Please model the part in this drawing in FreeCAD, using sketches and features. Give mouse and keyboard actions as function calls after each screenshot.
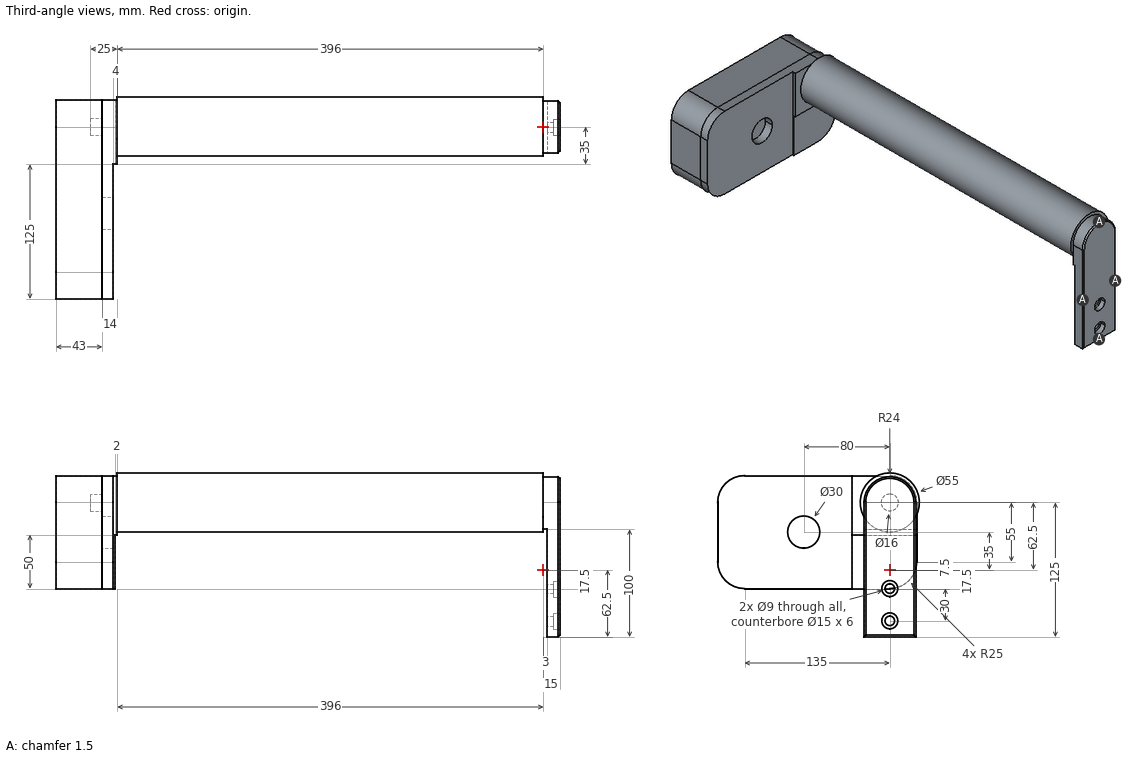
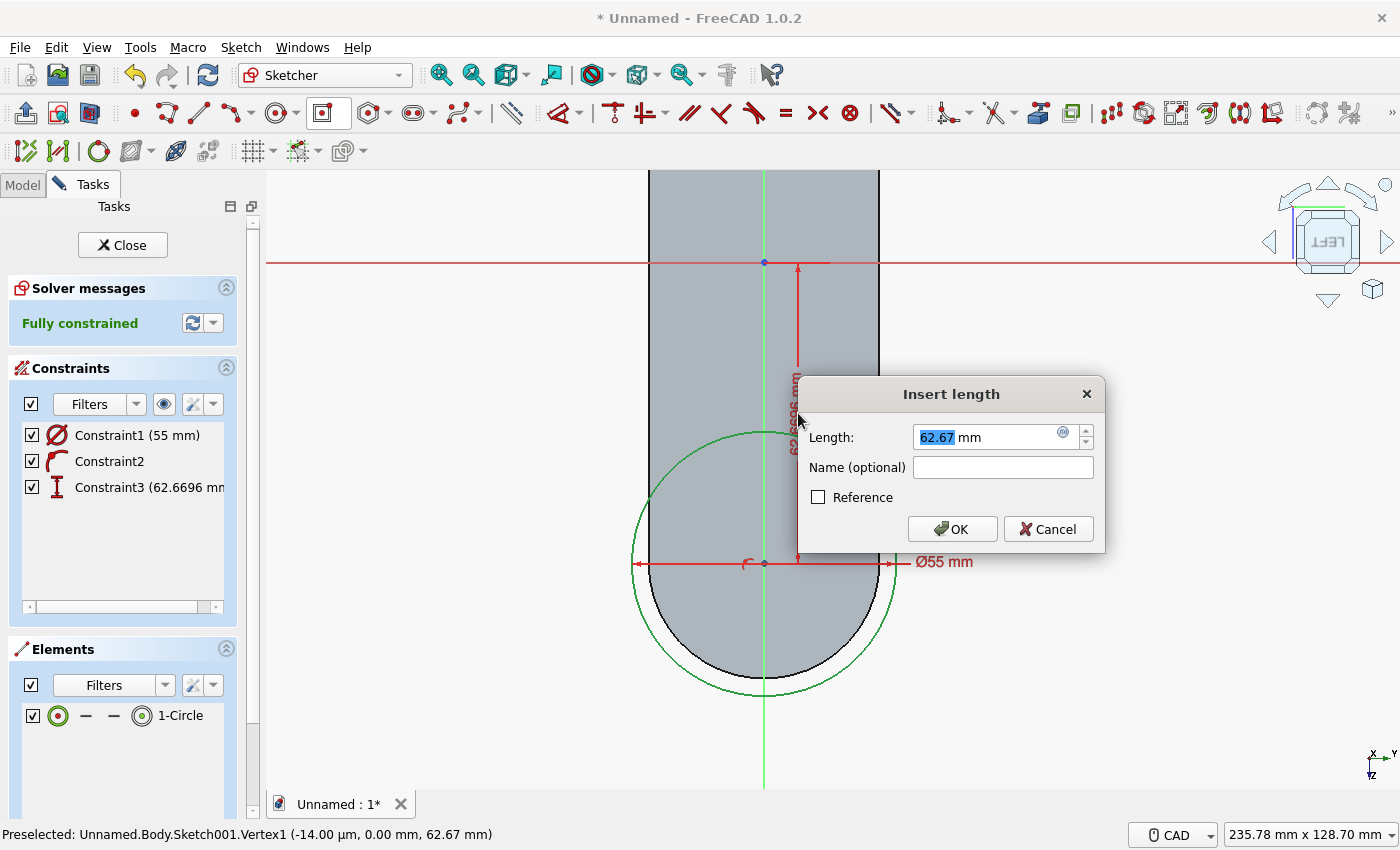
text(62.5)
key(Return)
key(Escape)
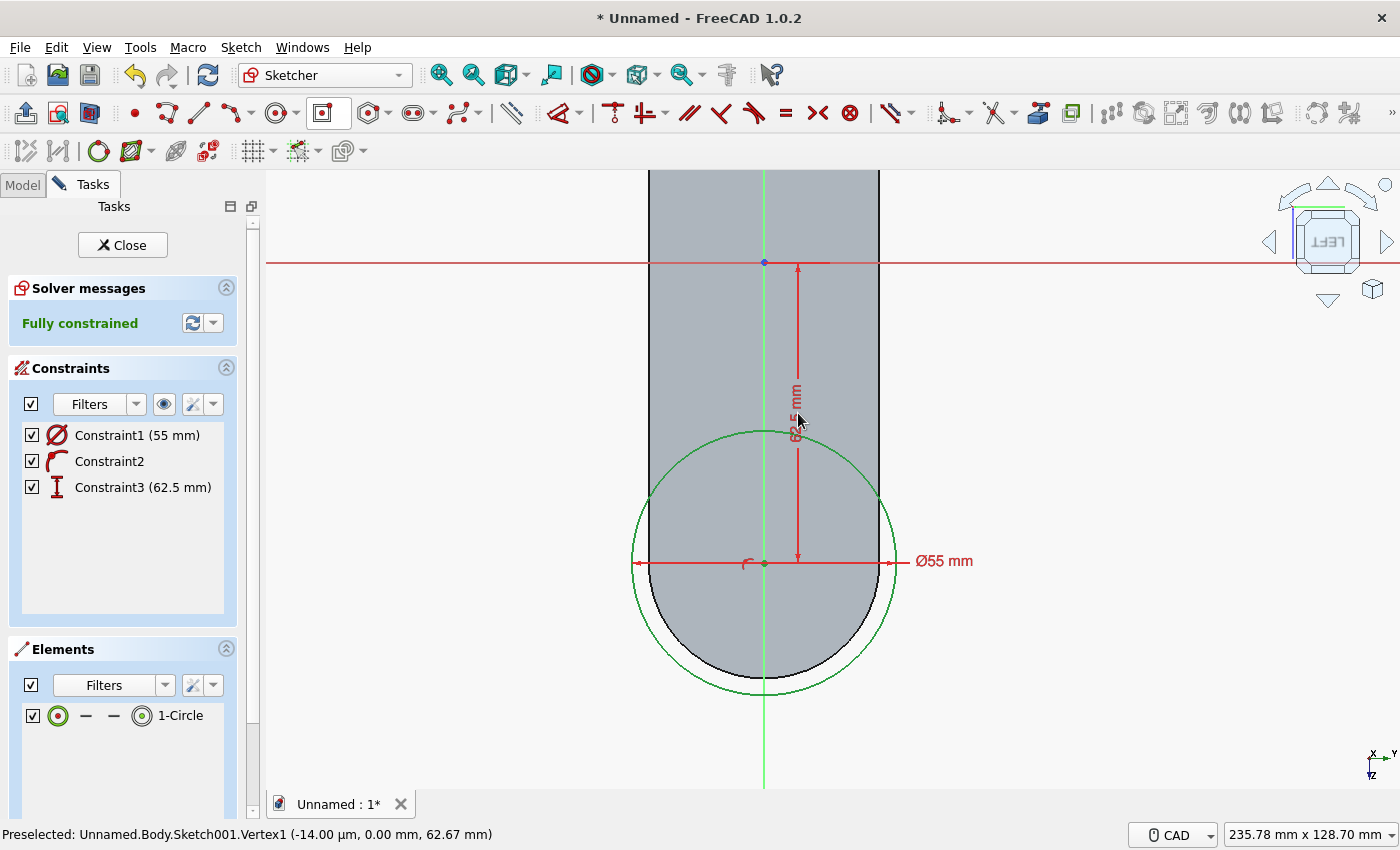
click(123, 245)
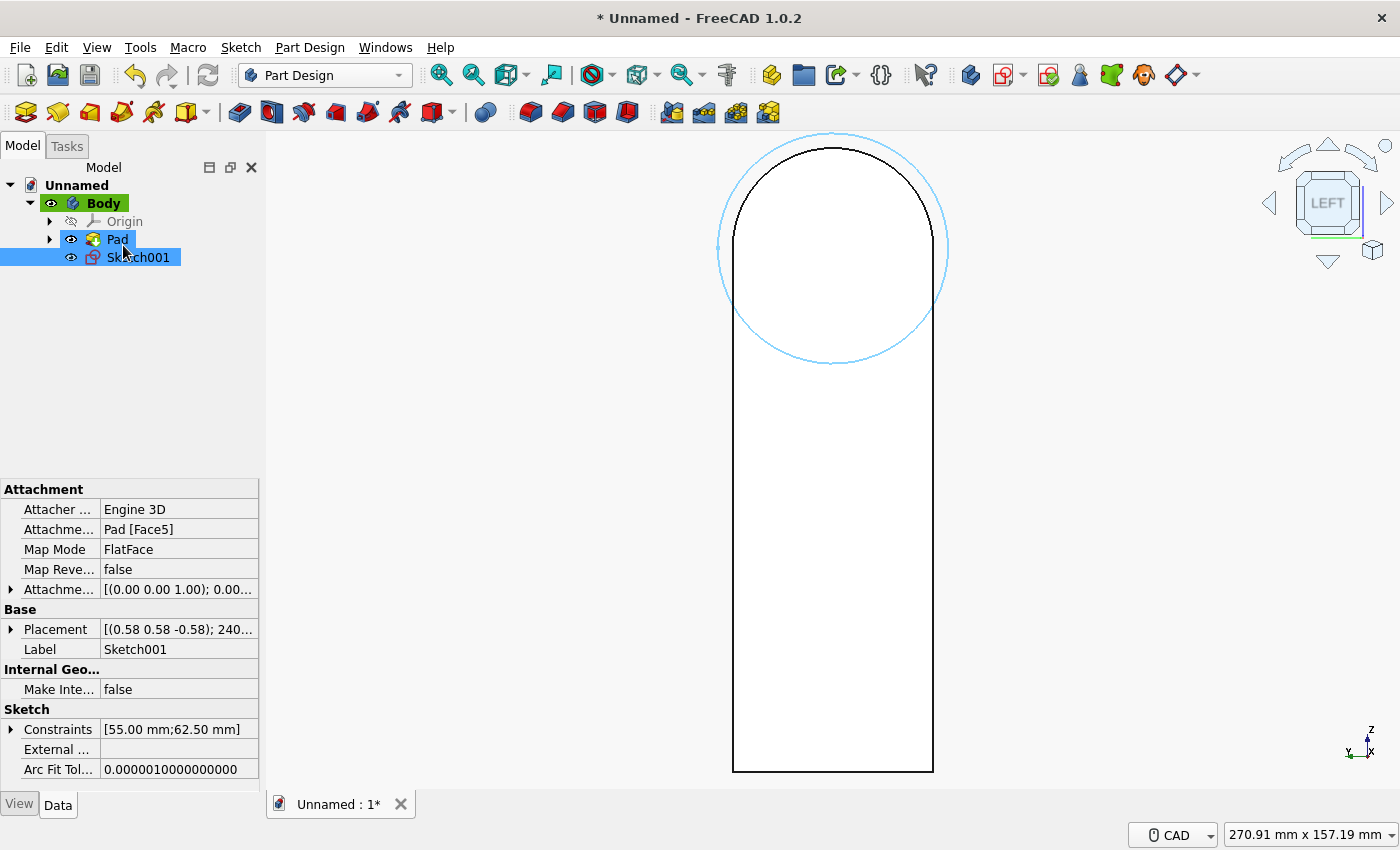
click(26, 112)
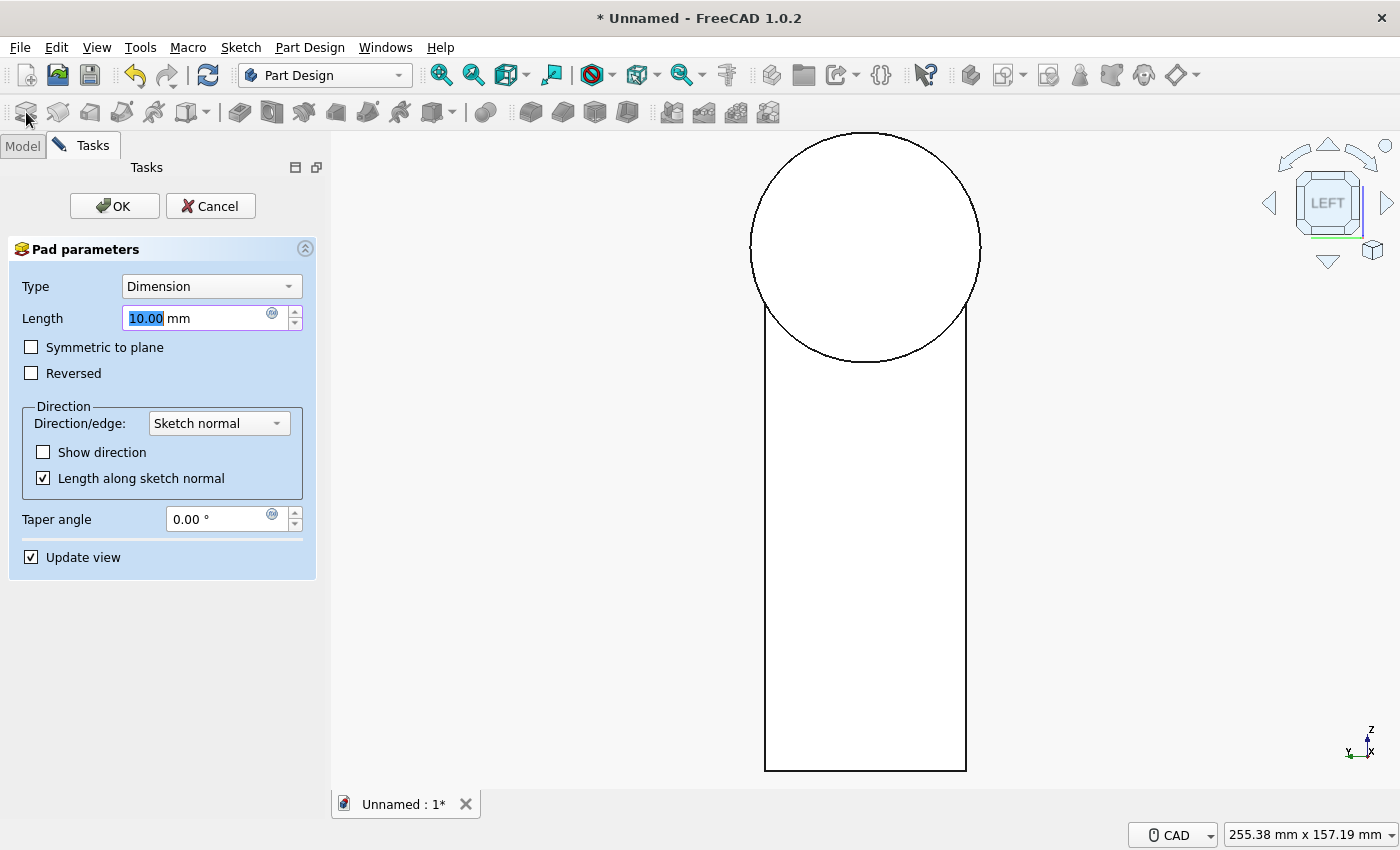
text(396)
key(Tab)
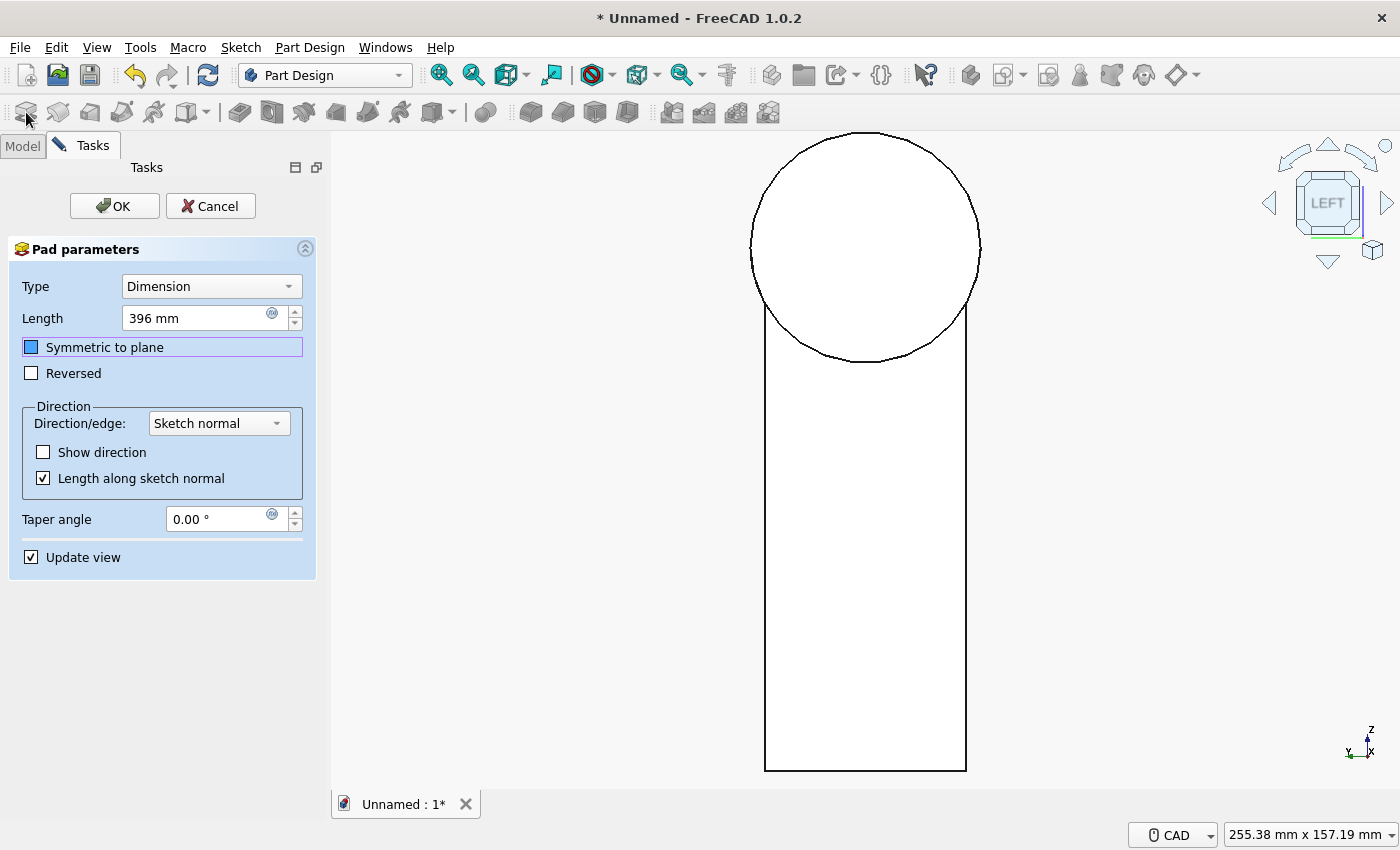
click(115, 206)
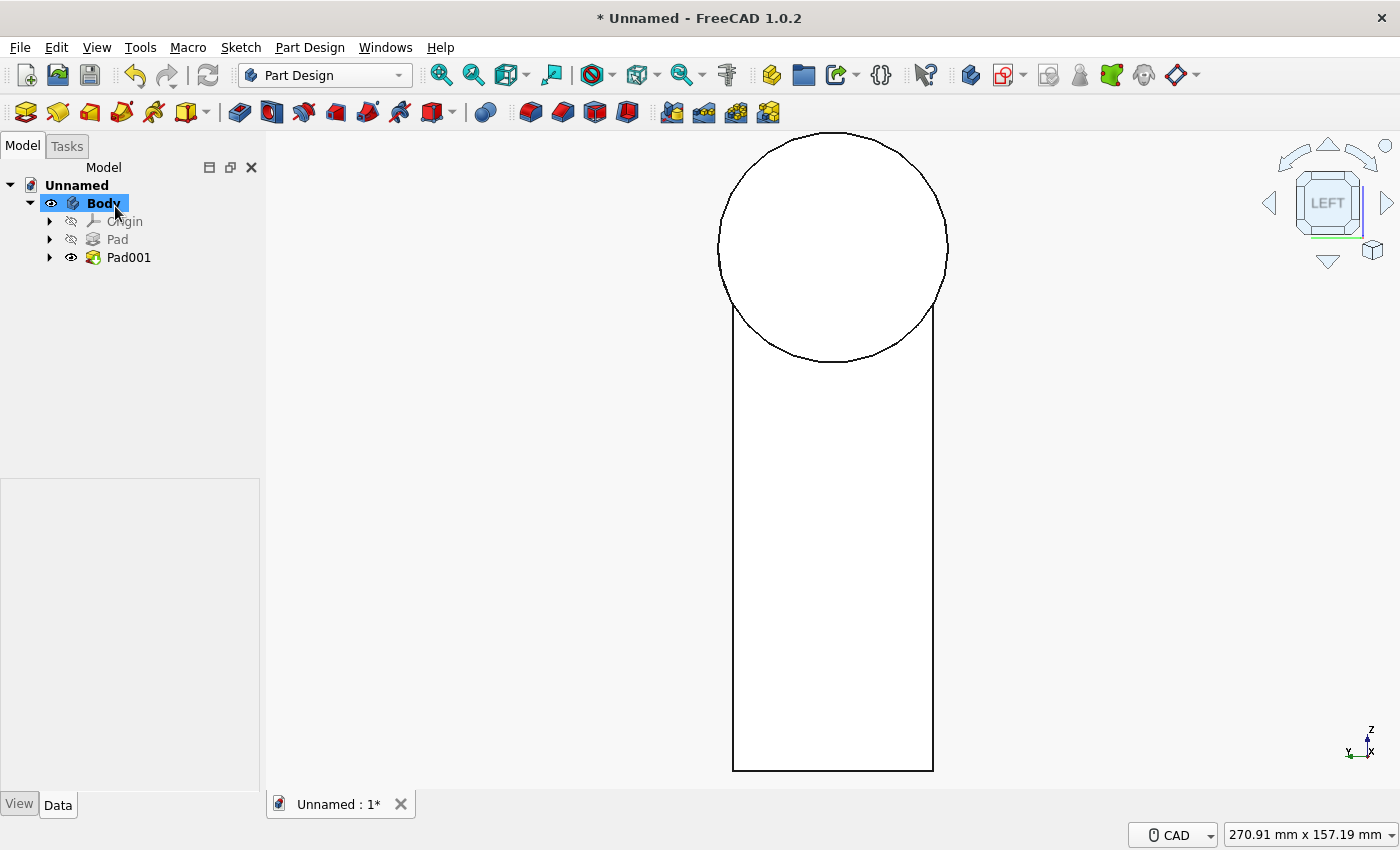
key(0)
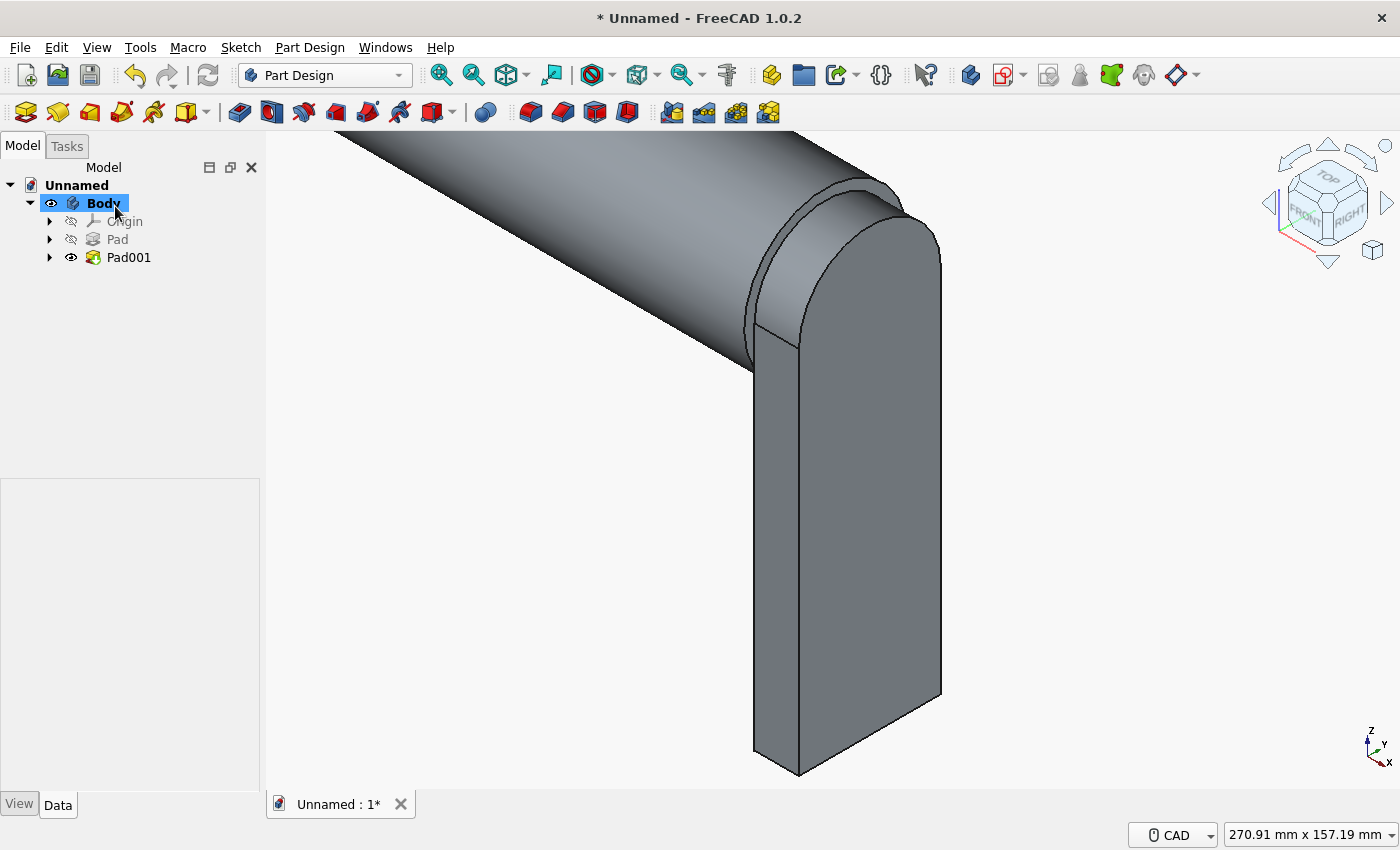
click(442, 76)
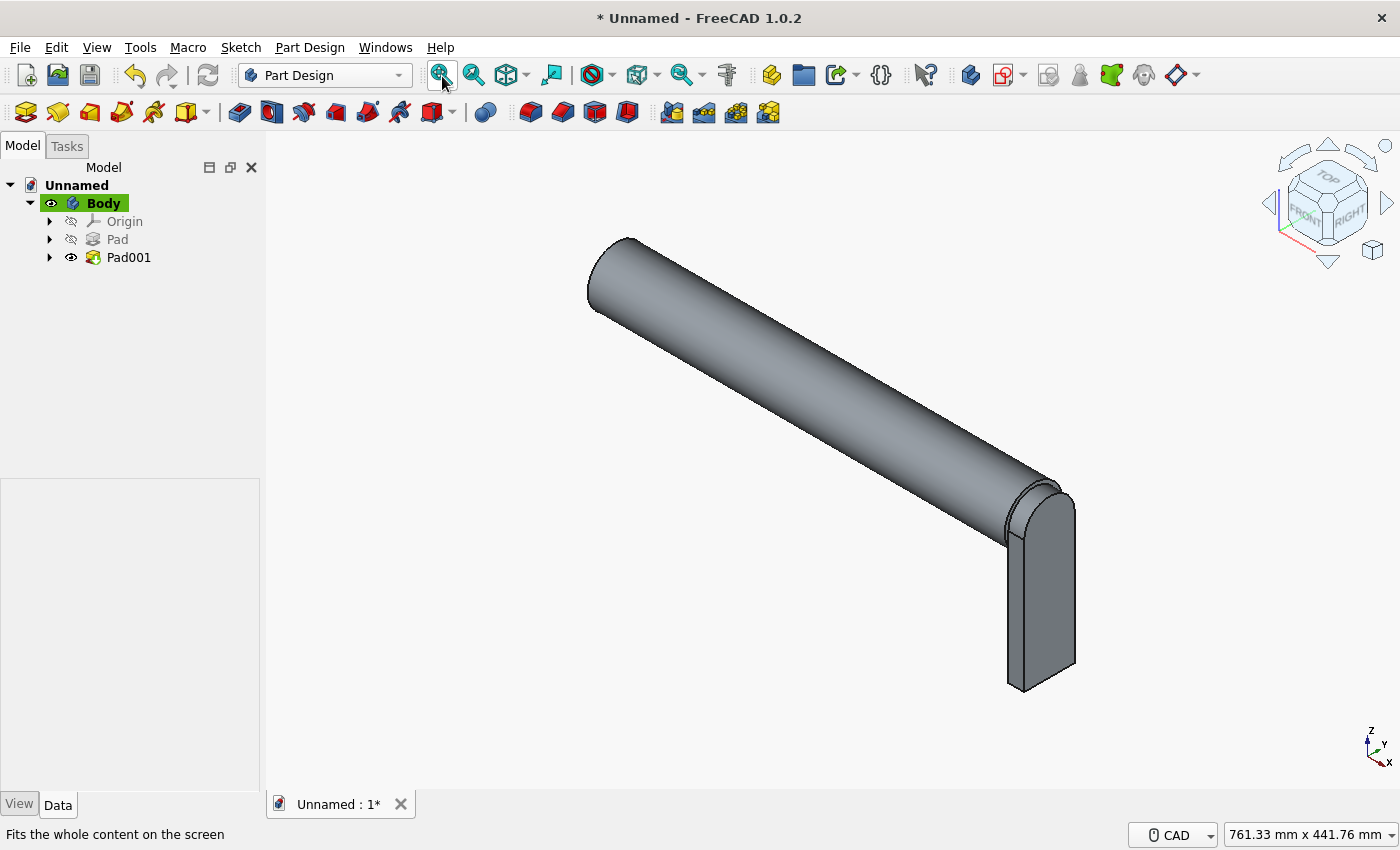
click(1049, 586)